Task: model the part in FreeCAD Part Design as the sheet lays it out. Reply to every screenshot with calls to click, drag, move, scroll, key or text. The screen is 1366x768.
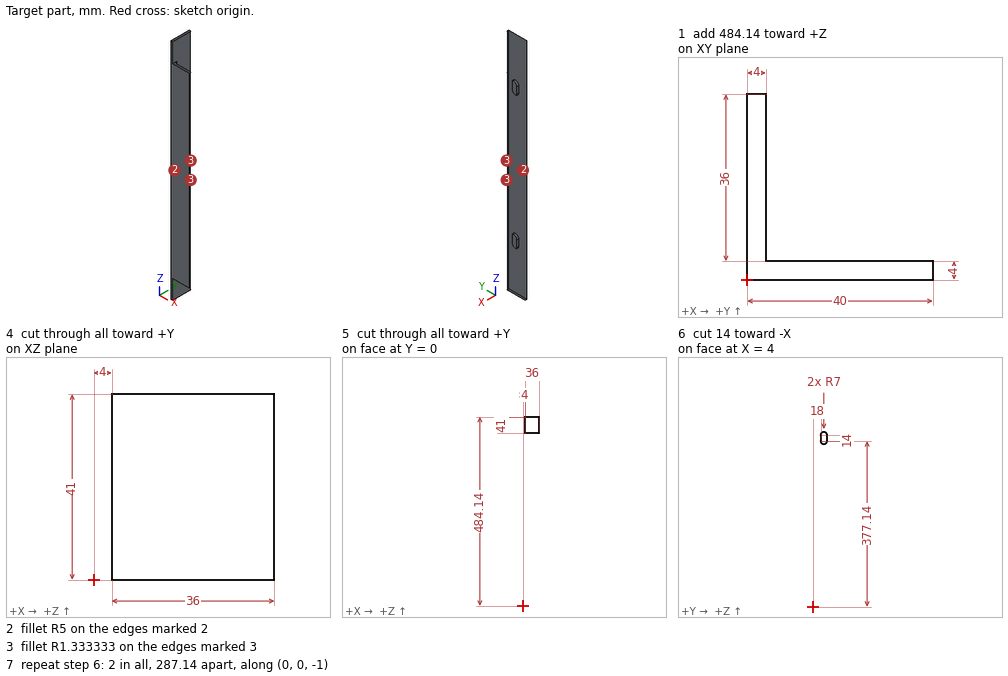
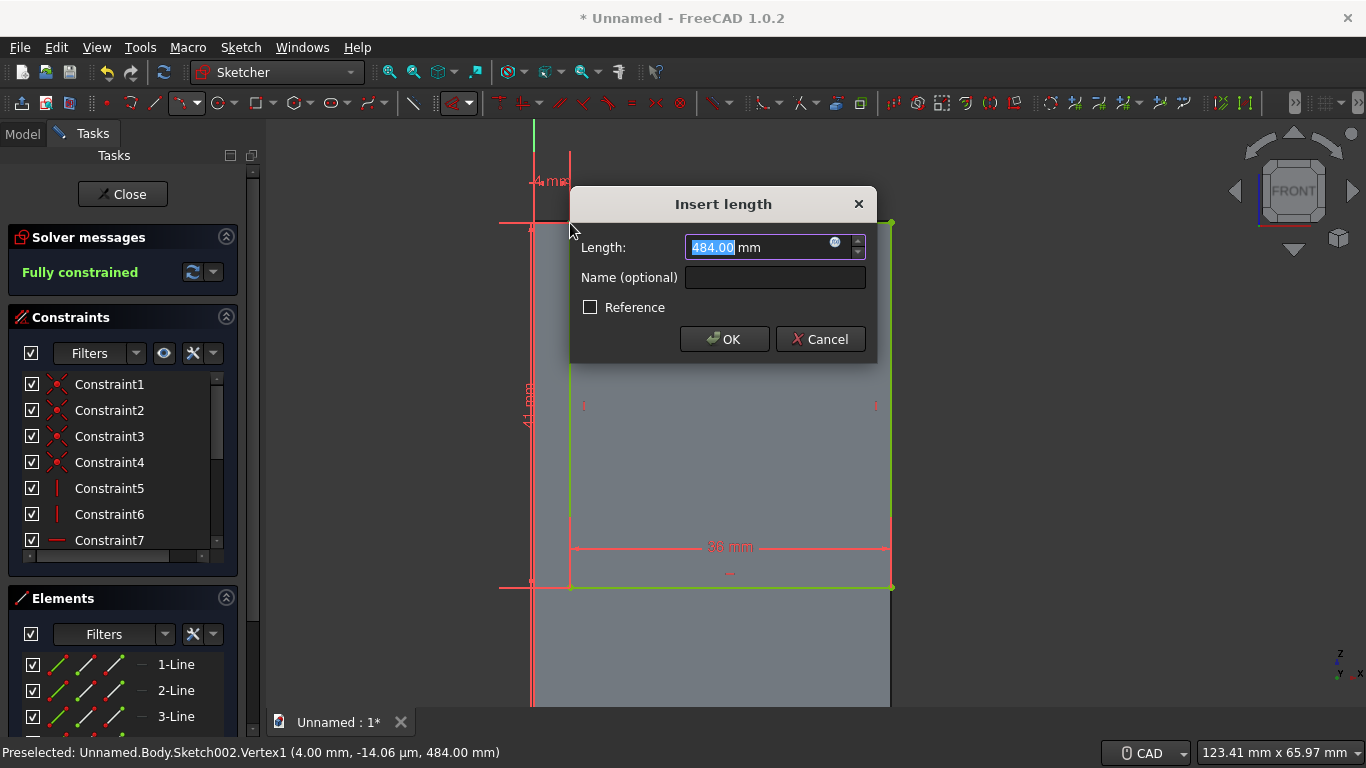
text(484.14)
key(Return)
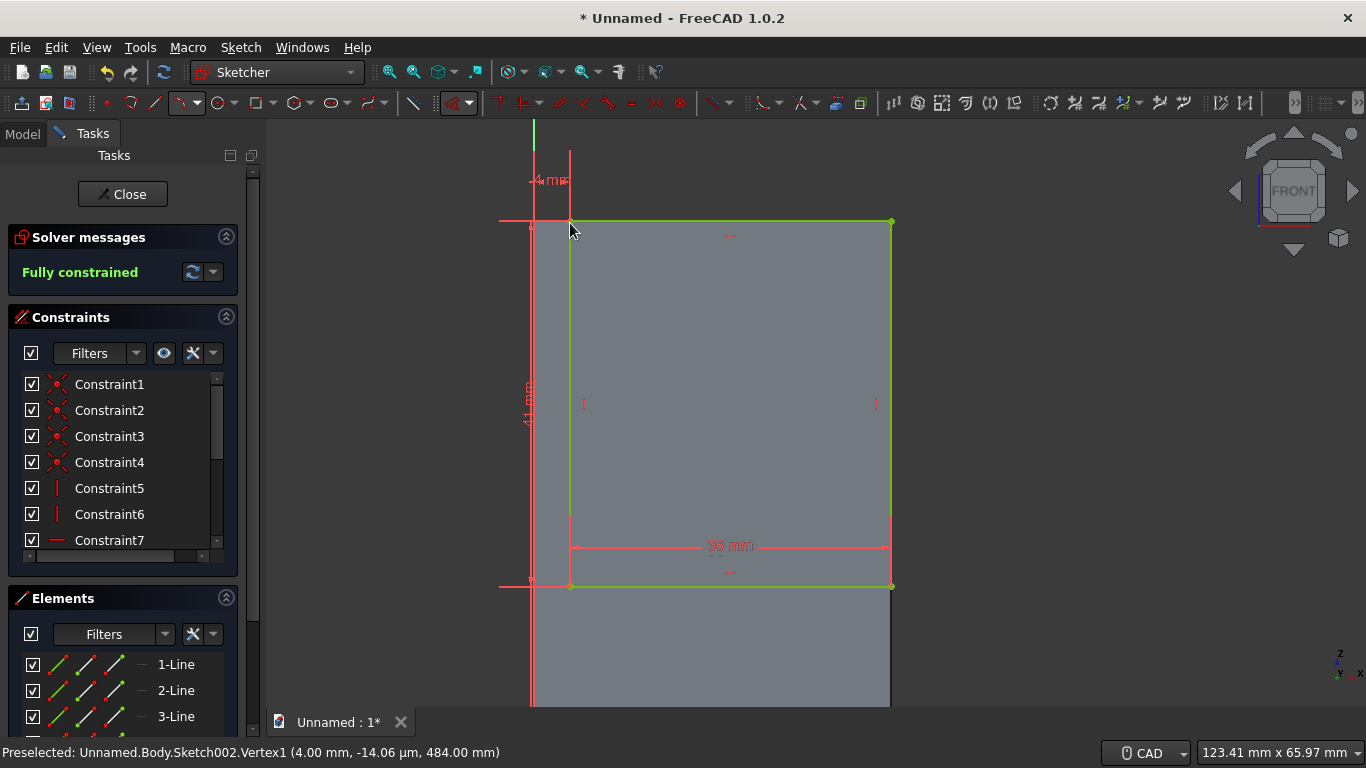
click(123, 194)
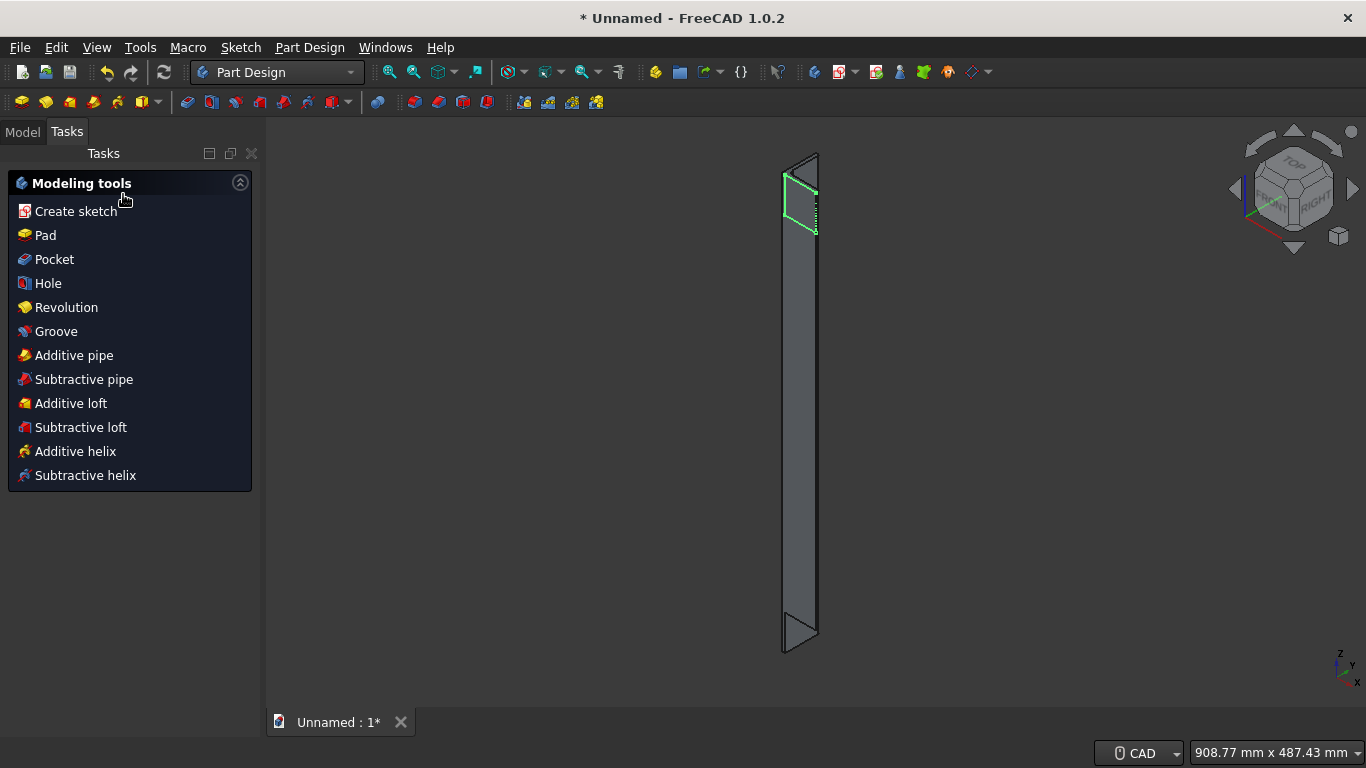
click(188, 102)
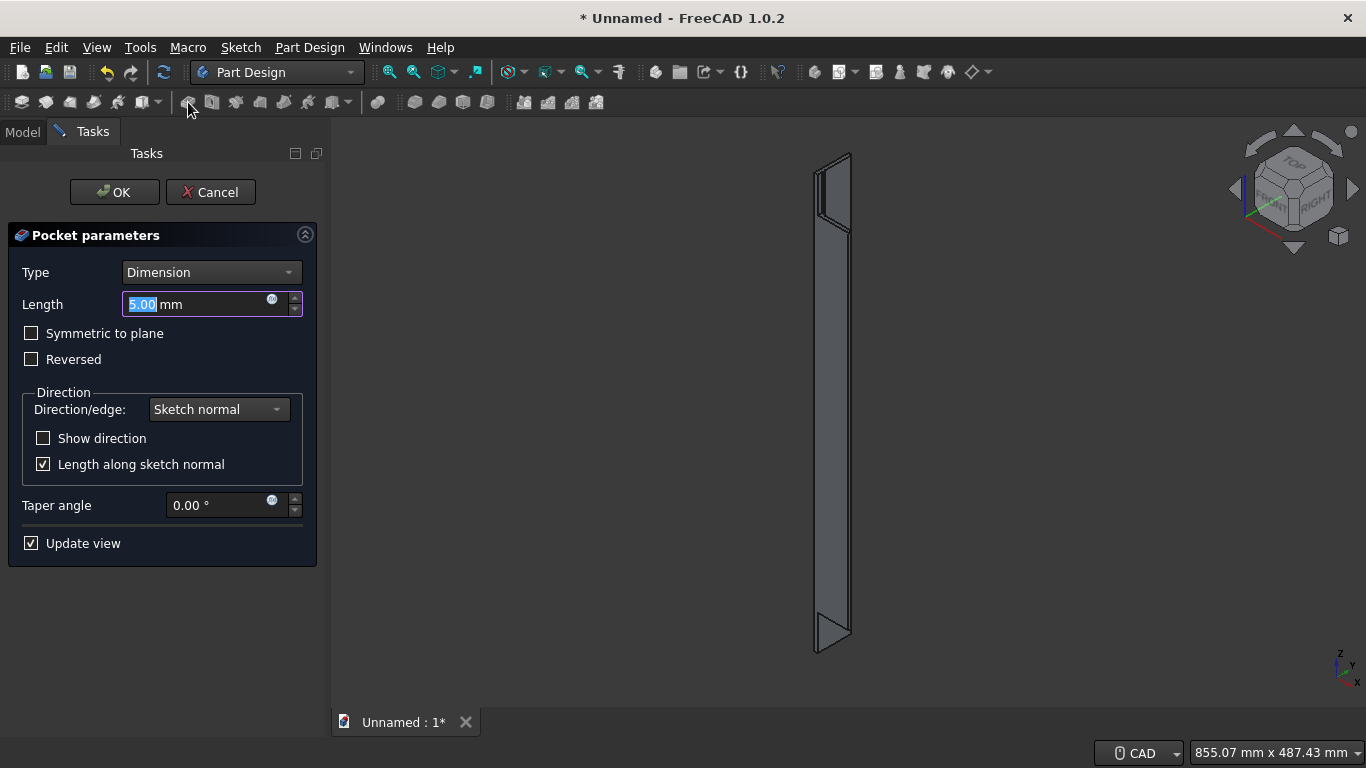
click(212, 272)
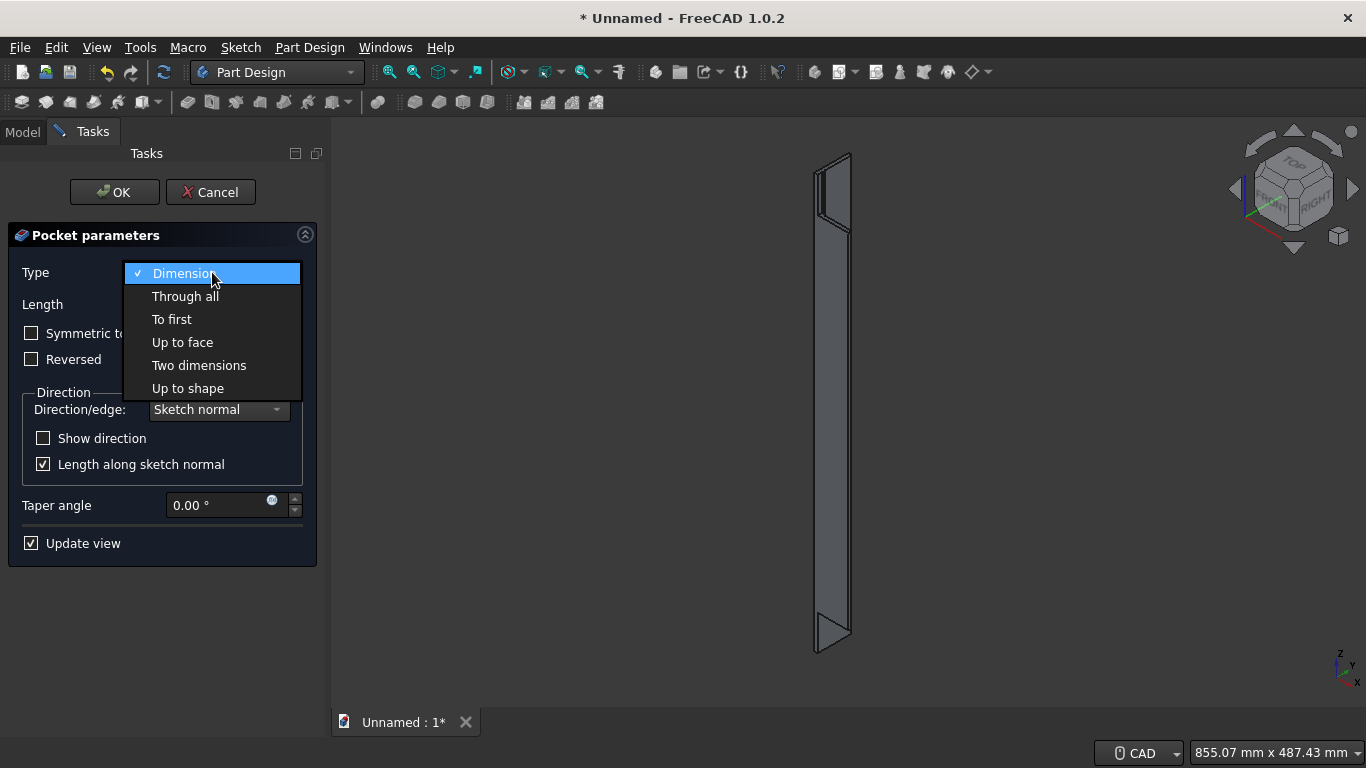
click(212, 296)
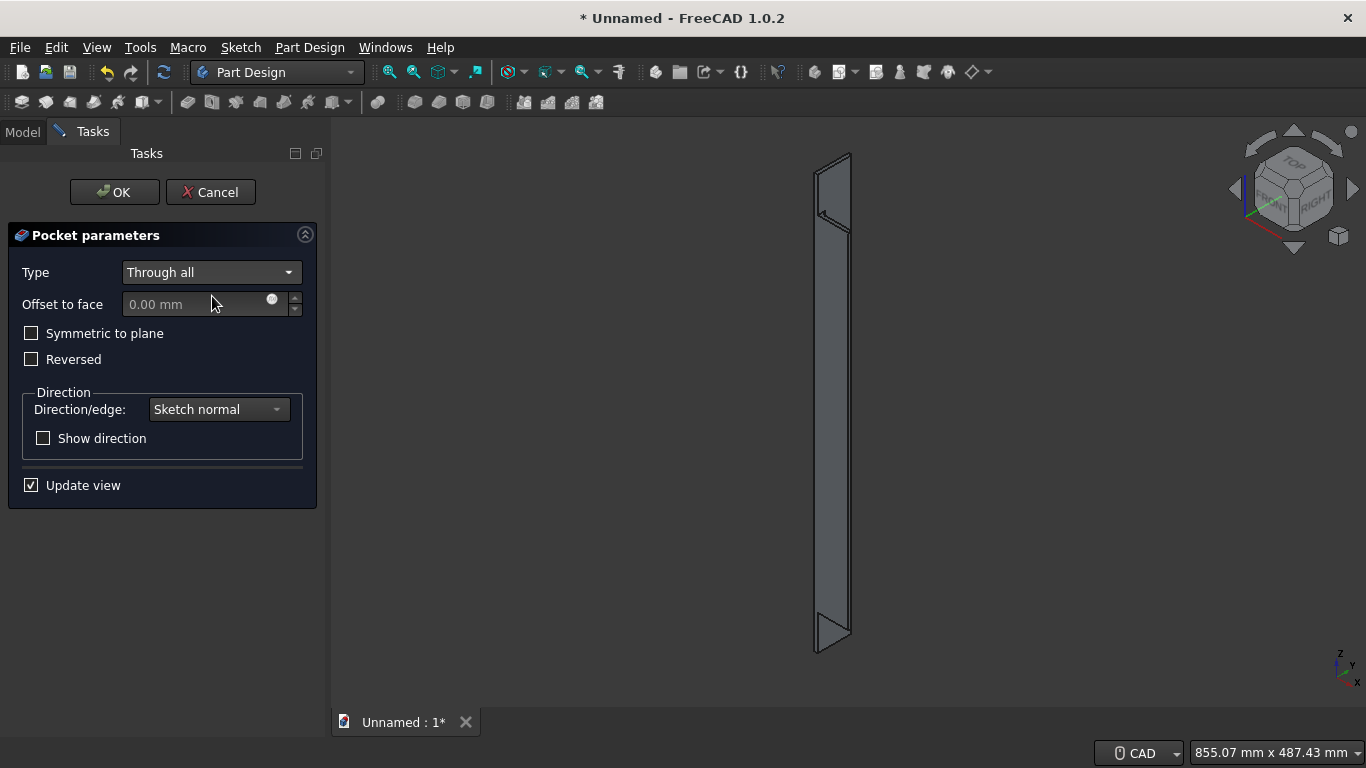
click(115, 192)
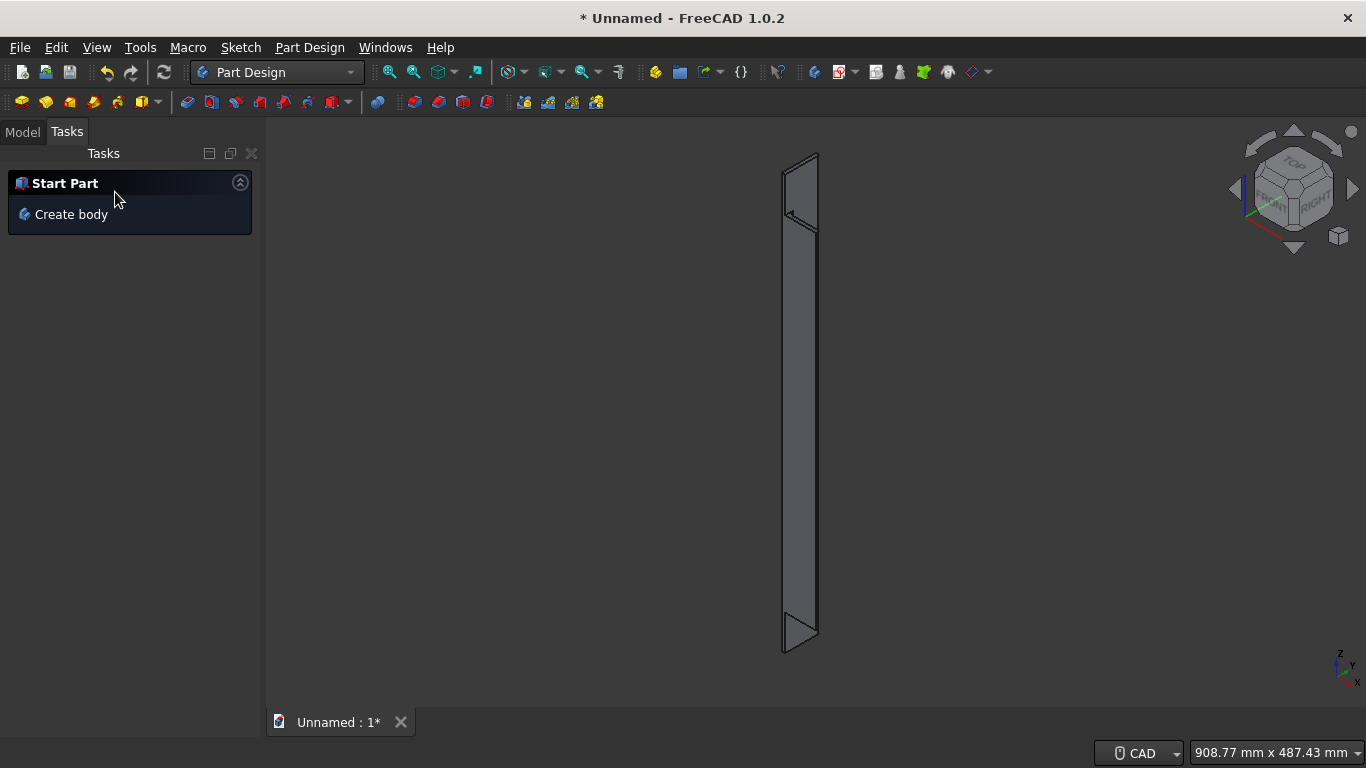
click(806, 196)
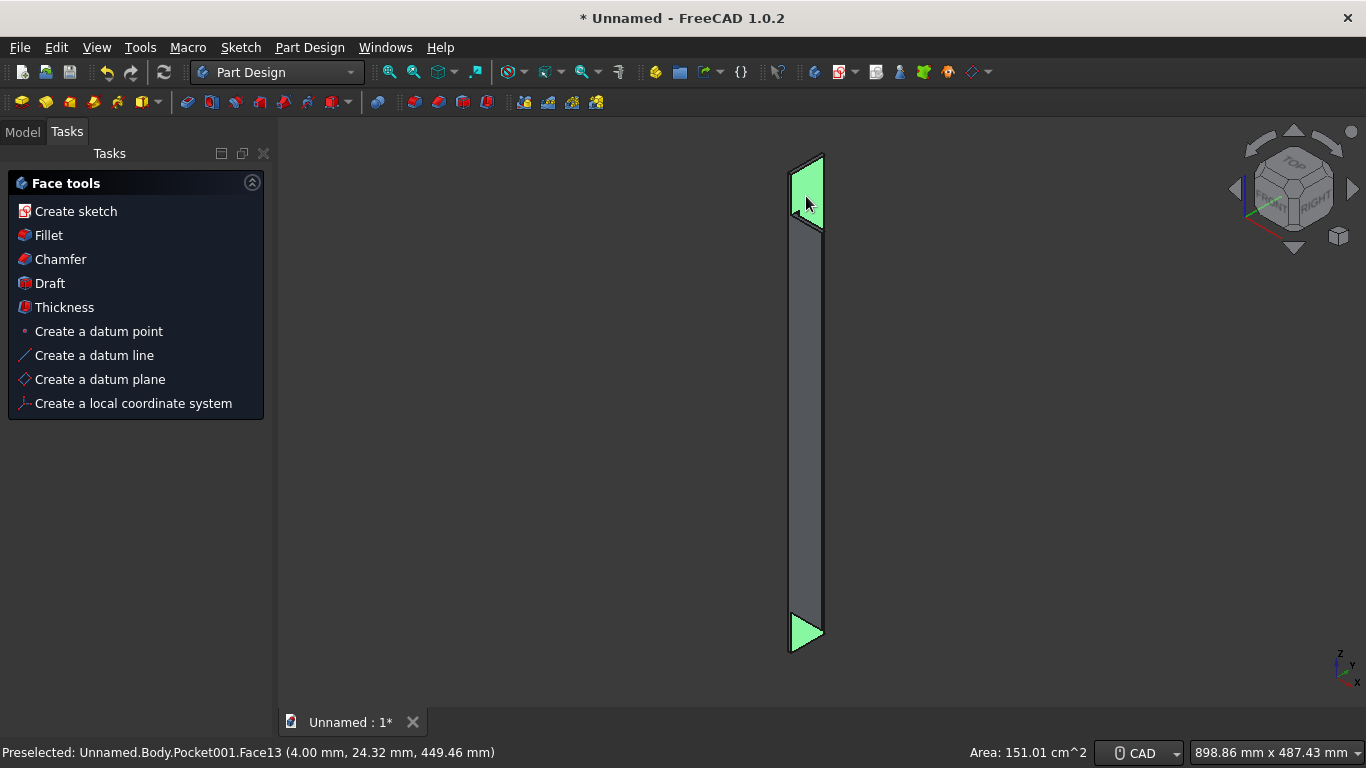
click(840, 72)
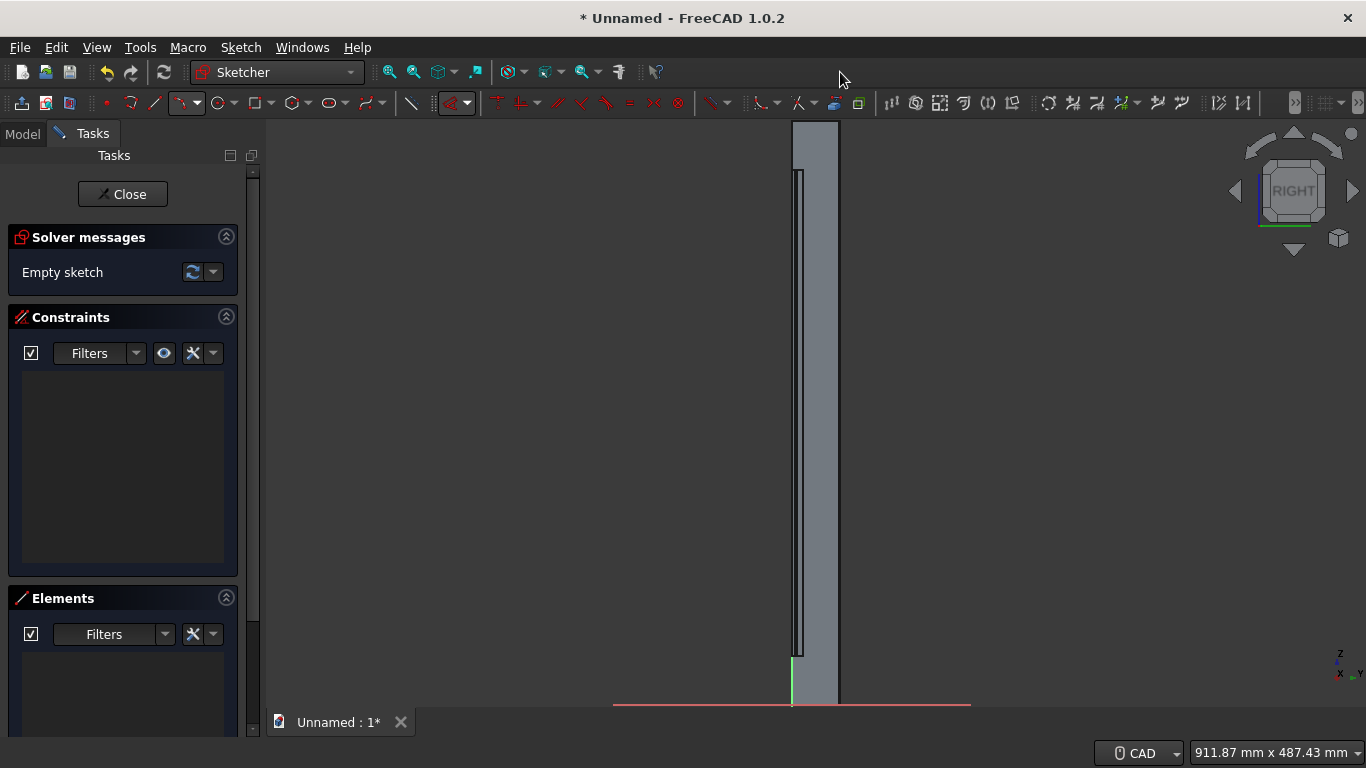
click(70, 104)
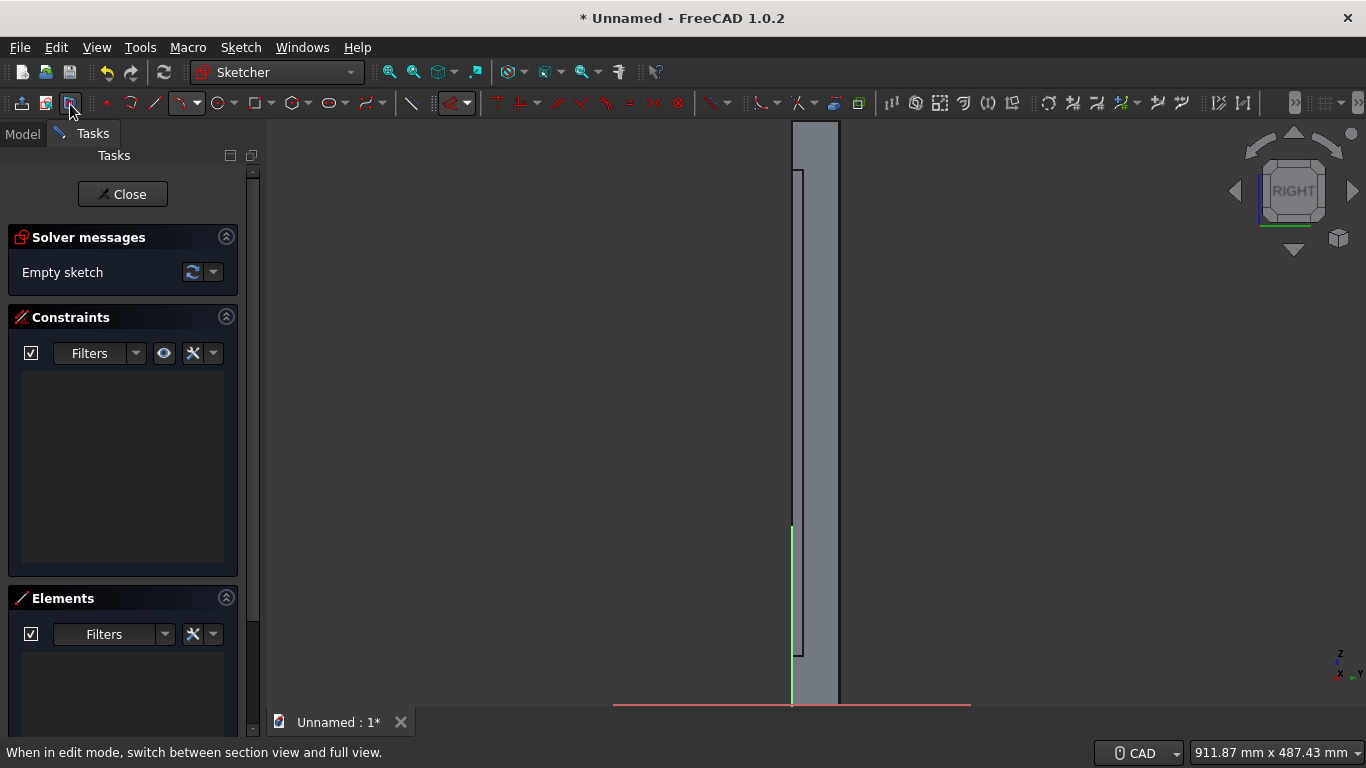
scroll(829, 225, up, 12)